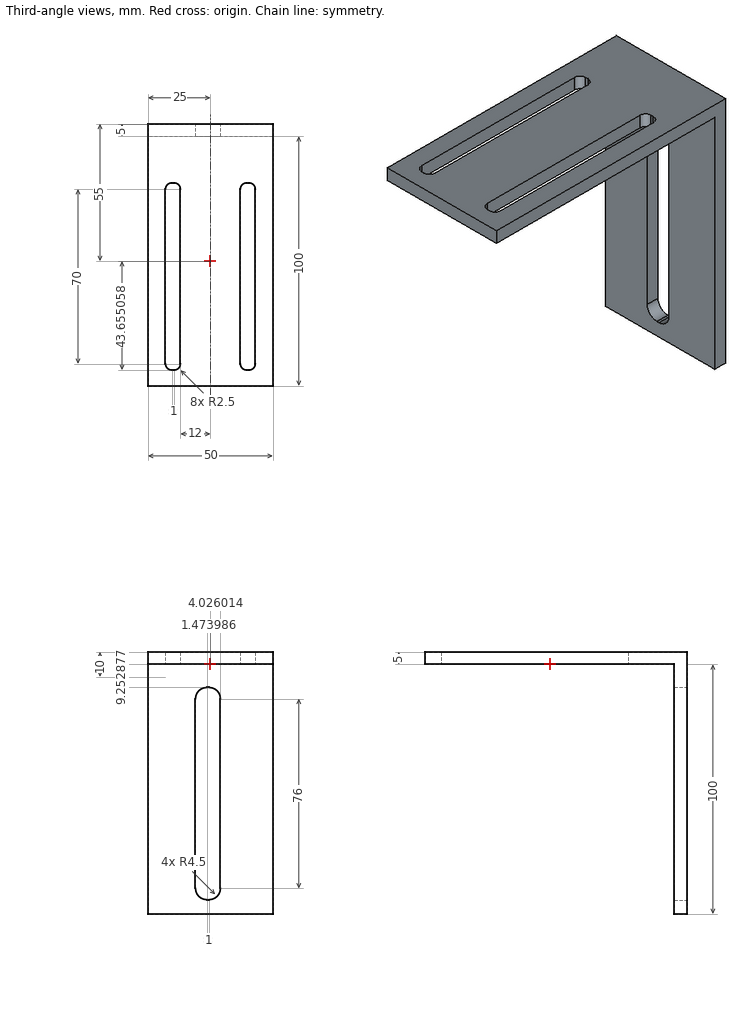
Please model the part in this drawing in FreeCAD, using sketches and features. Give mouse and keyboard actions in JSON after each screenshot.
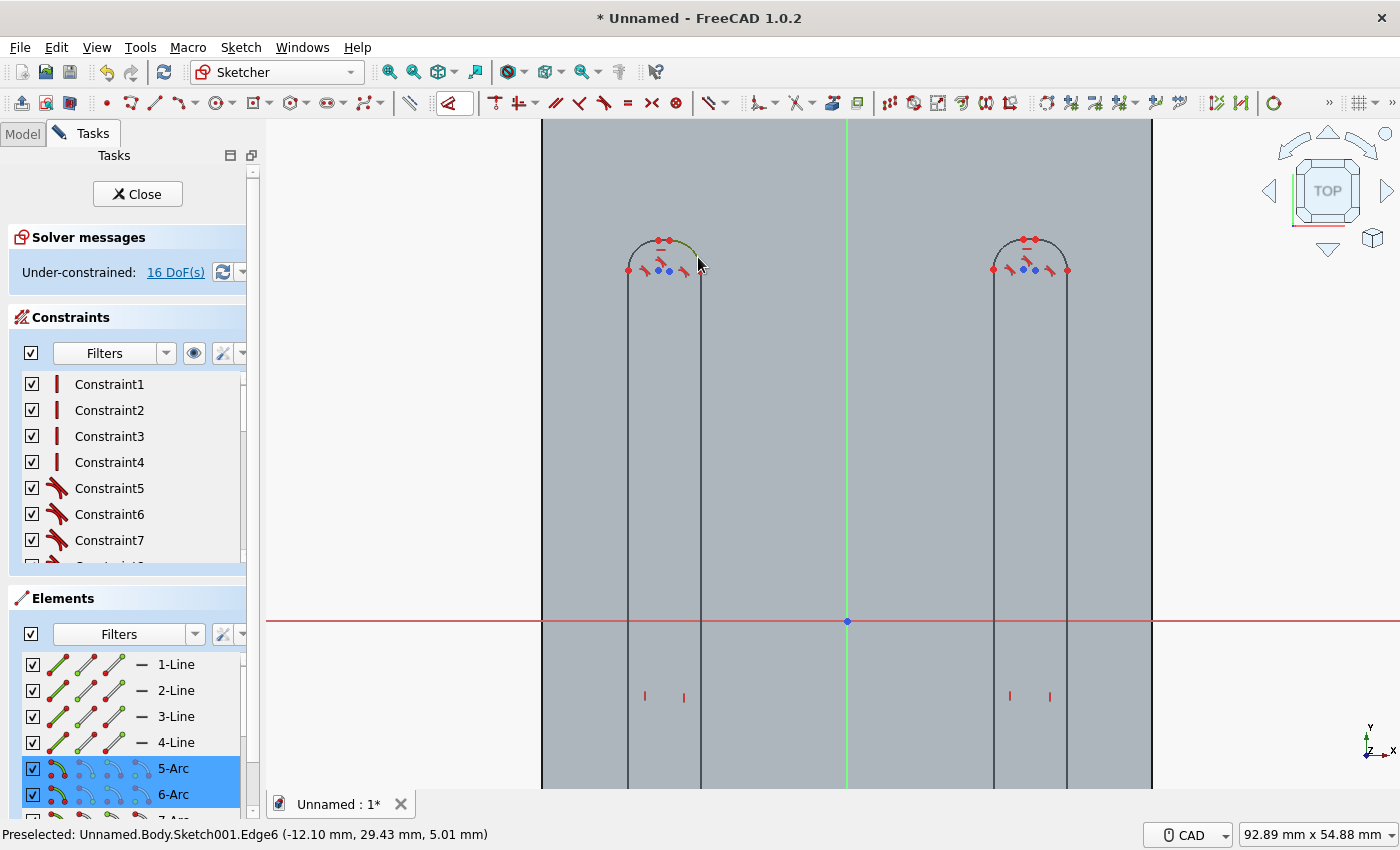
{"action": "left_click", "coordinate": [645, 244]}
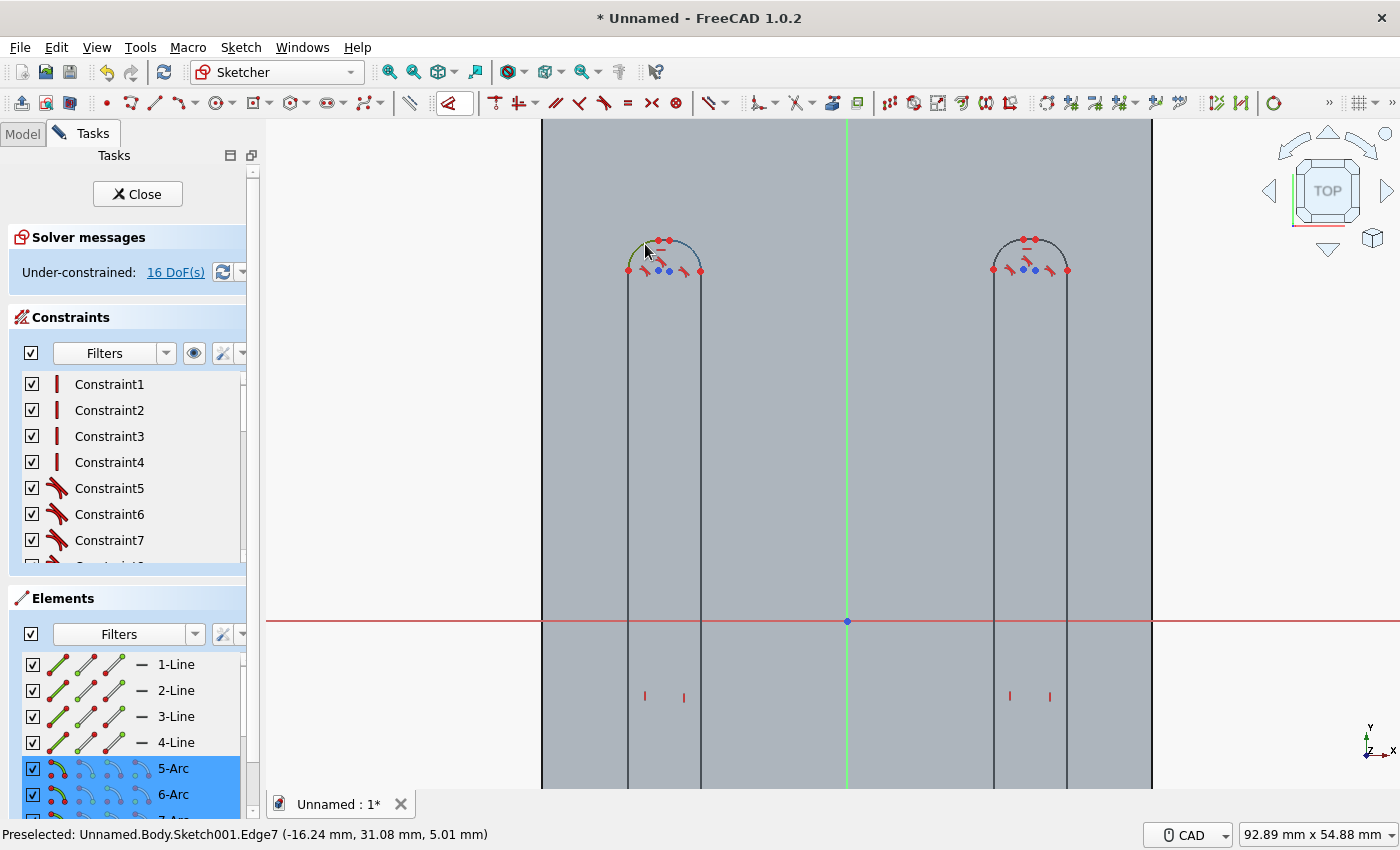
{"action": "scroll", "coordinate": [697, 256], "scroll_direction": "down", "scroll_amount": 4}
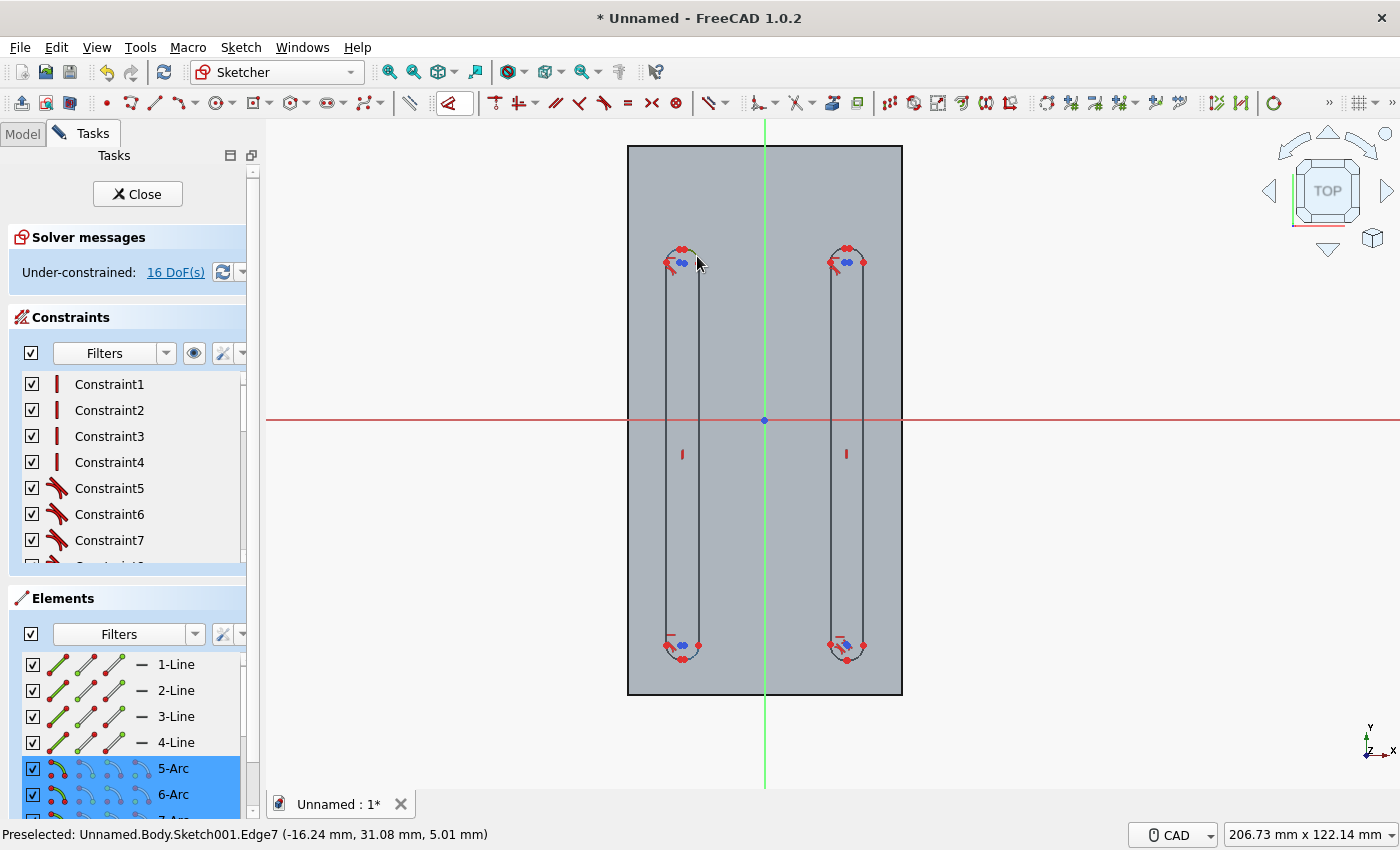
{"action": "scroll", "coordinate": [668, 652], "scroll_direction": "up", "scroll_amount": 4}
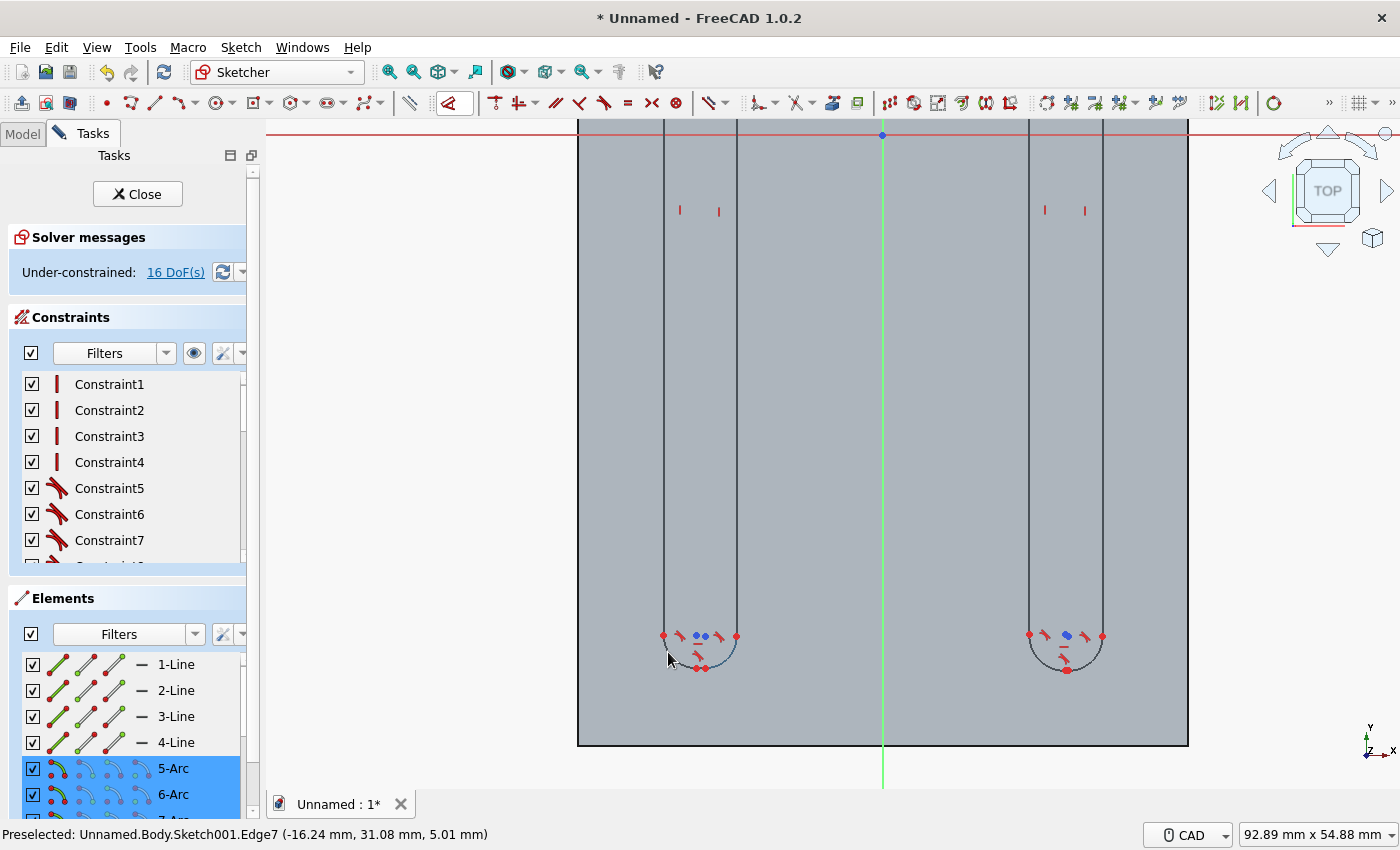
{"action": "left_click", "coordinate": [667, 650]}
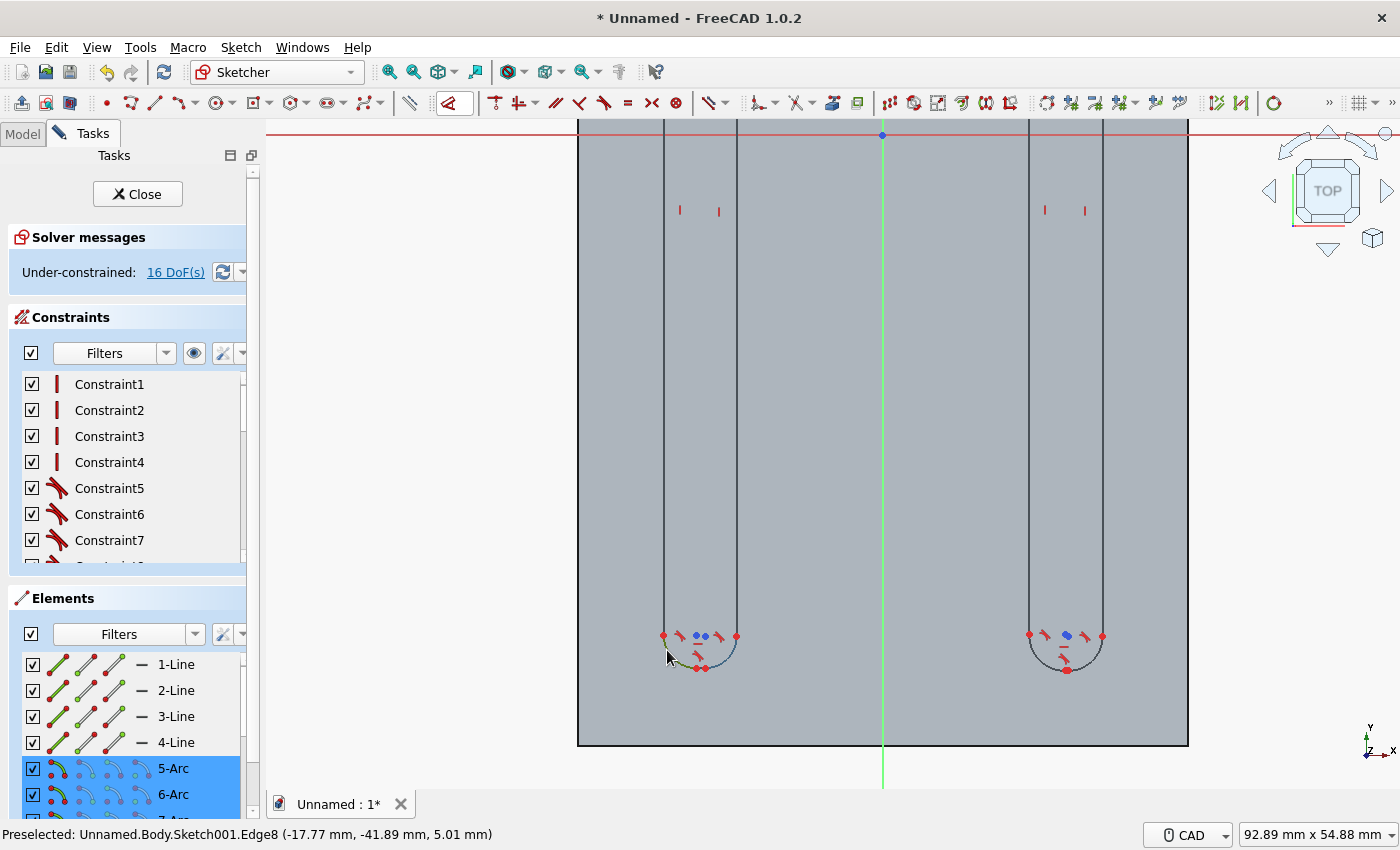
{"action": "left_click", "coordinate": [1084, 667]}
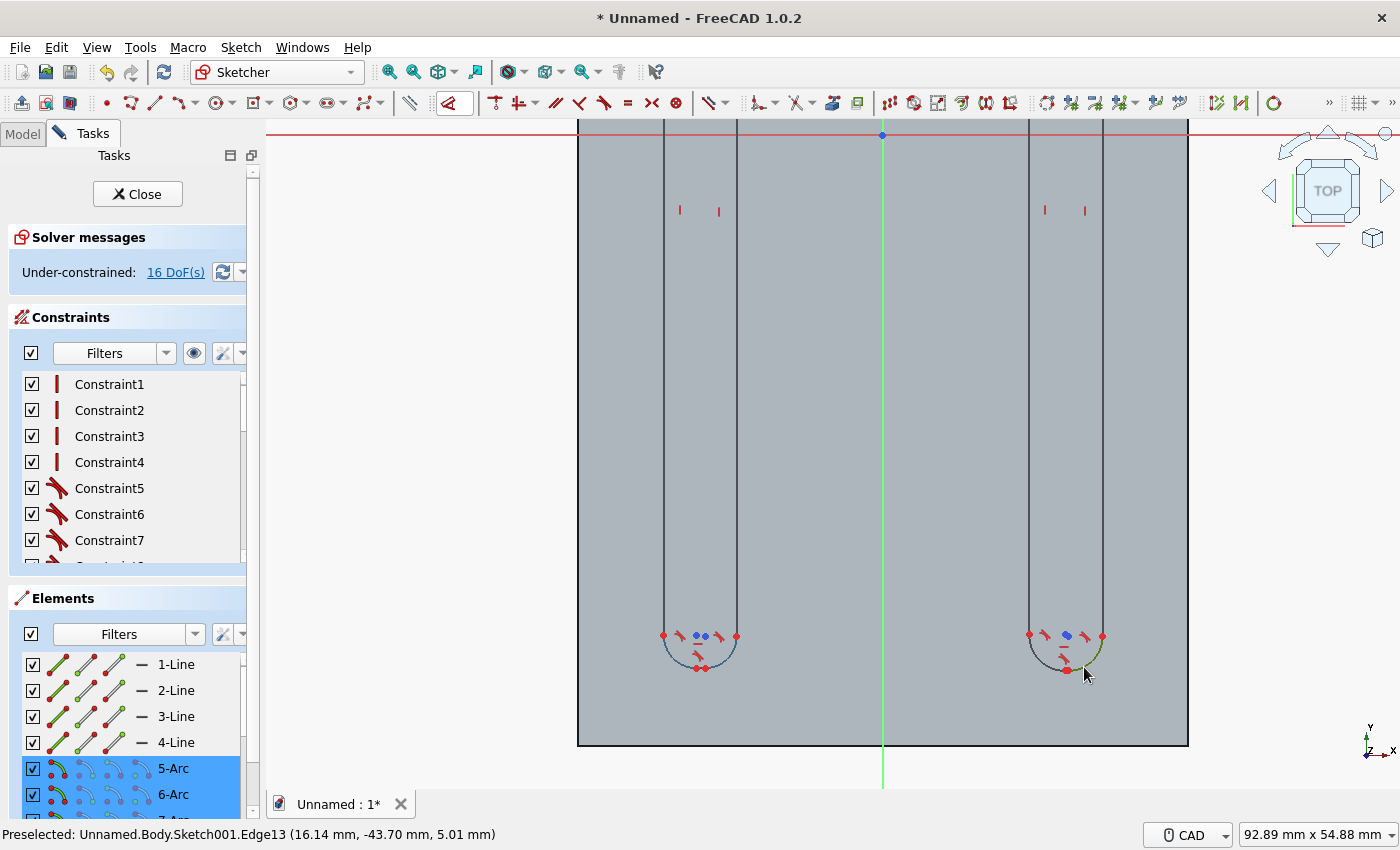
{"action": "scroll", "coordinate": [668, 653], "scroll_direction": "down", "scroll_amount": 4}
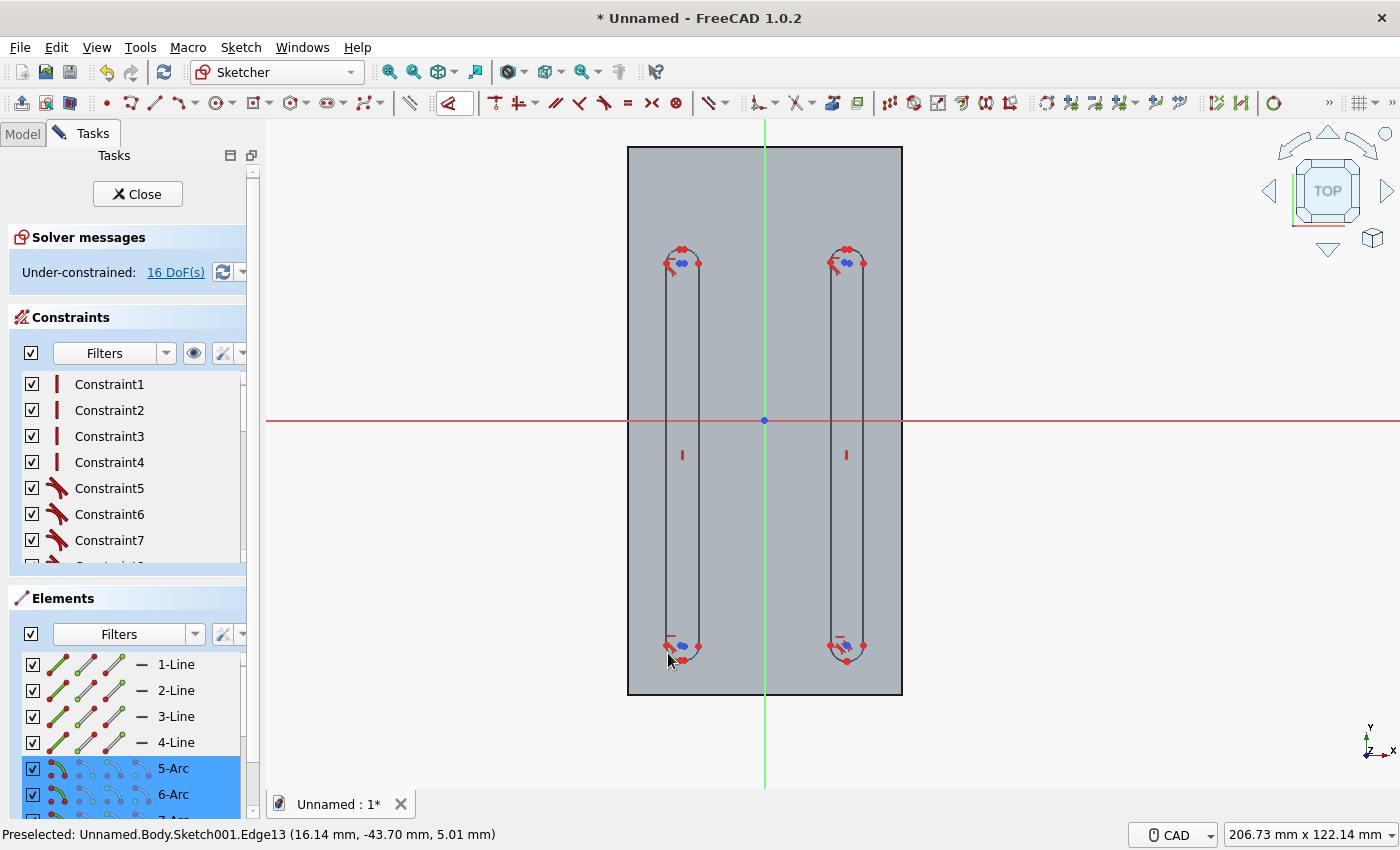
{"action": "scroll", "coordinate": [862, 257], "scroll_direction": "up", "scroll_amount": 4}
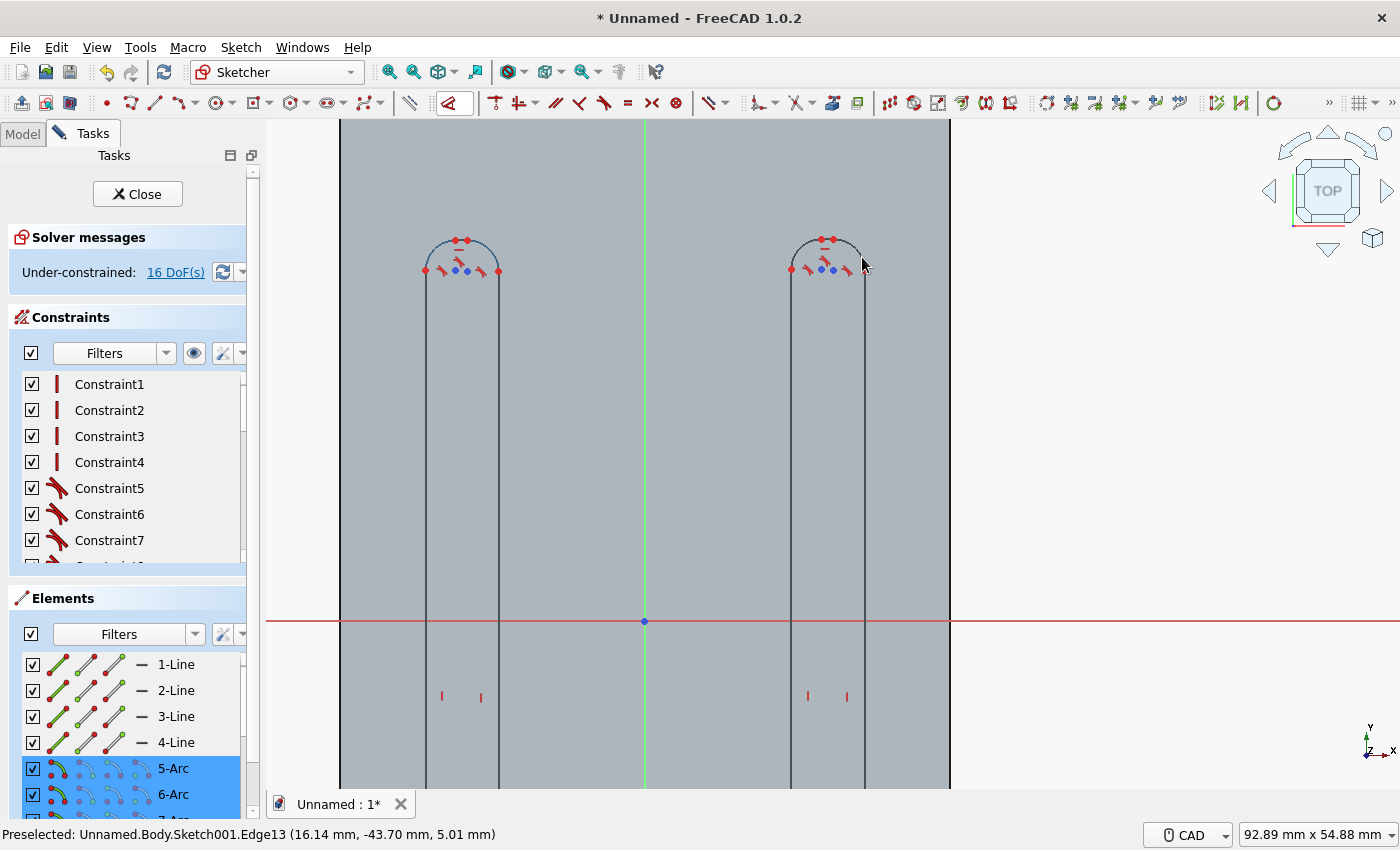
{"action": "left_click", "coordinate": [861, 256]}